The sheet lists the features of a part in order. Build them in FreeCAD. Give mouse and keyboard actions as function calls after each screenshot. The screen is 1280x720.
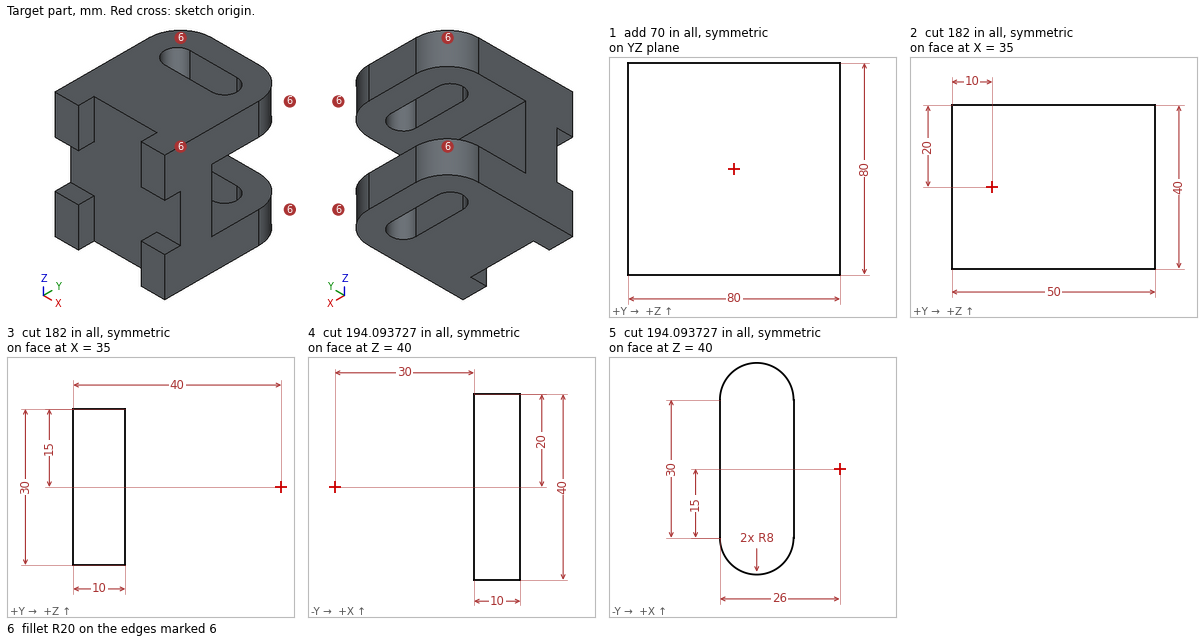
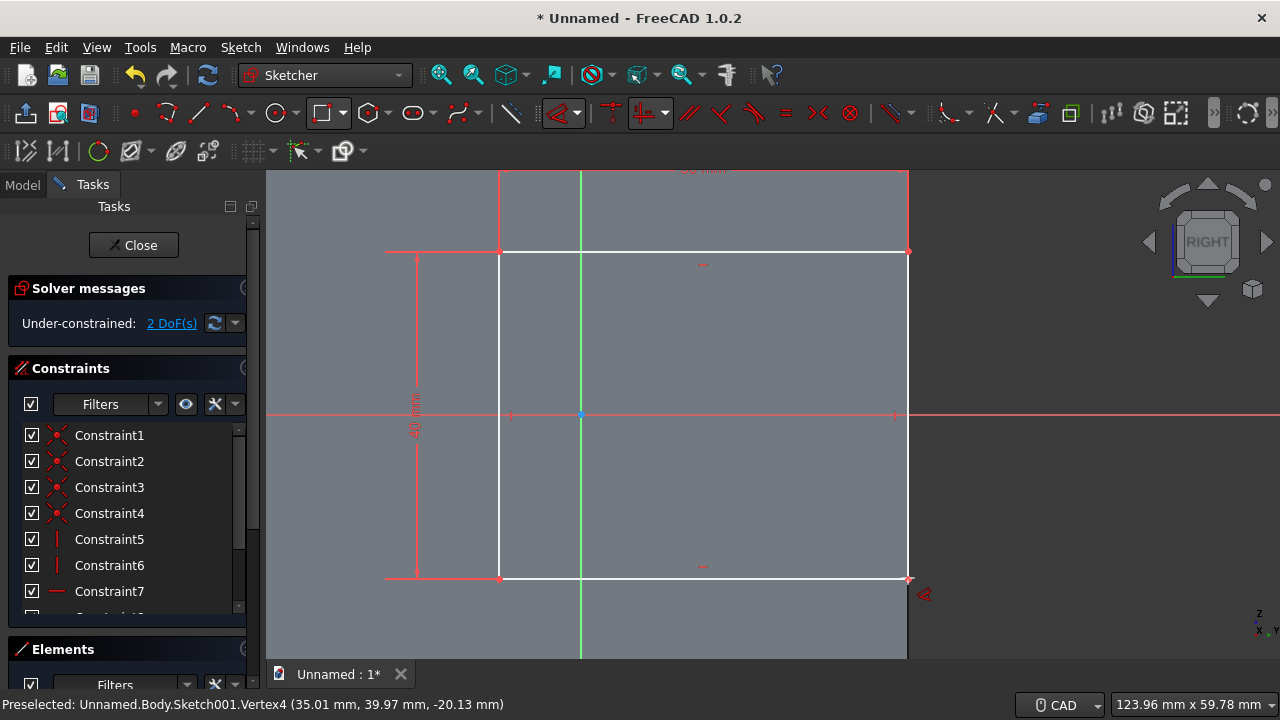
click(499, 252)
click(540, 218)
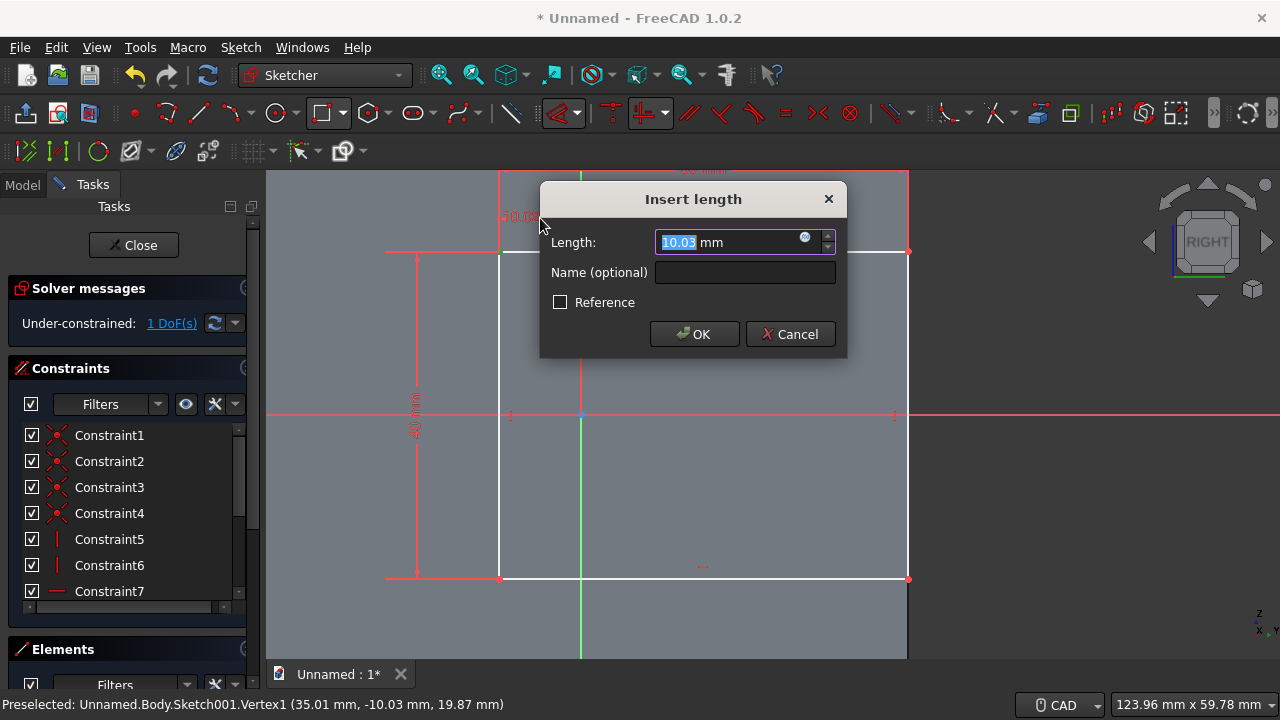
text(10)
key(Return)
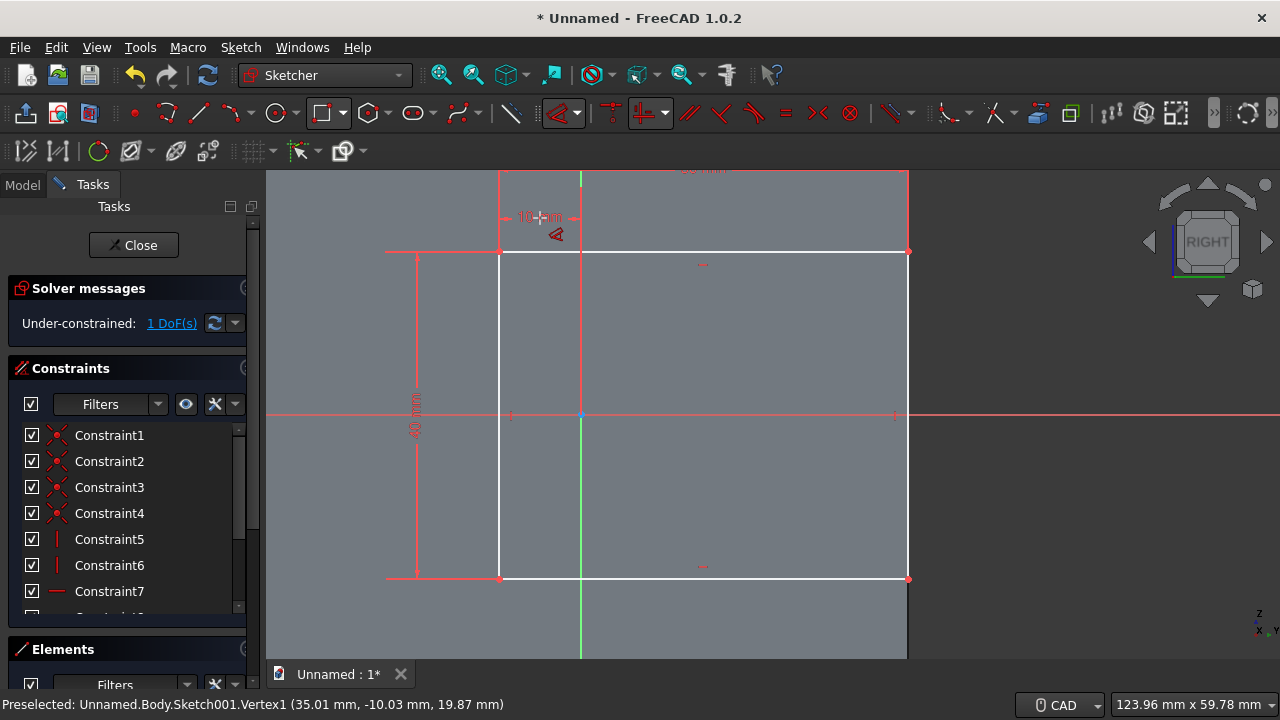
click(499, 252)
click(465, 333)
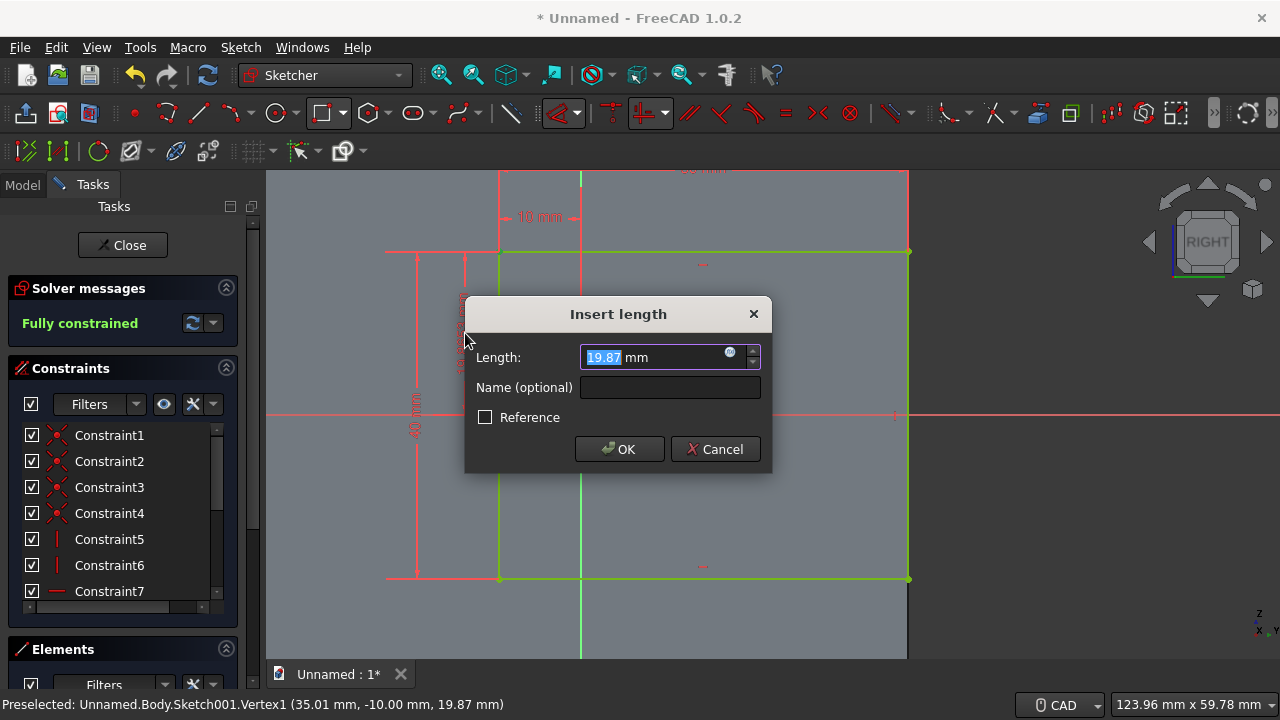
text(20)
key(Return)
key(Escape)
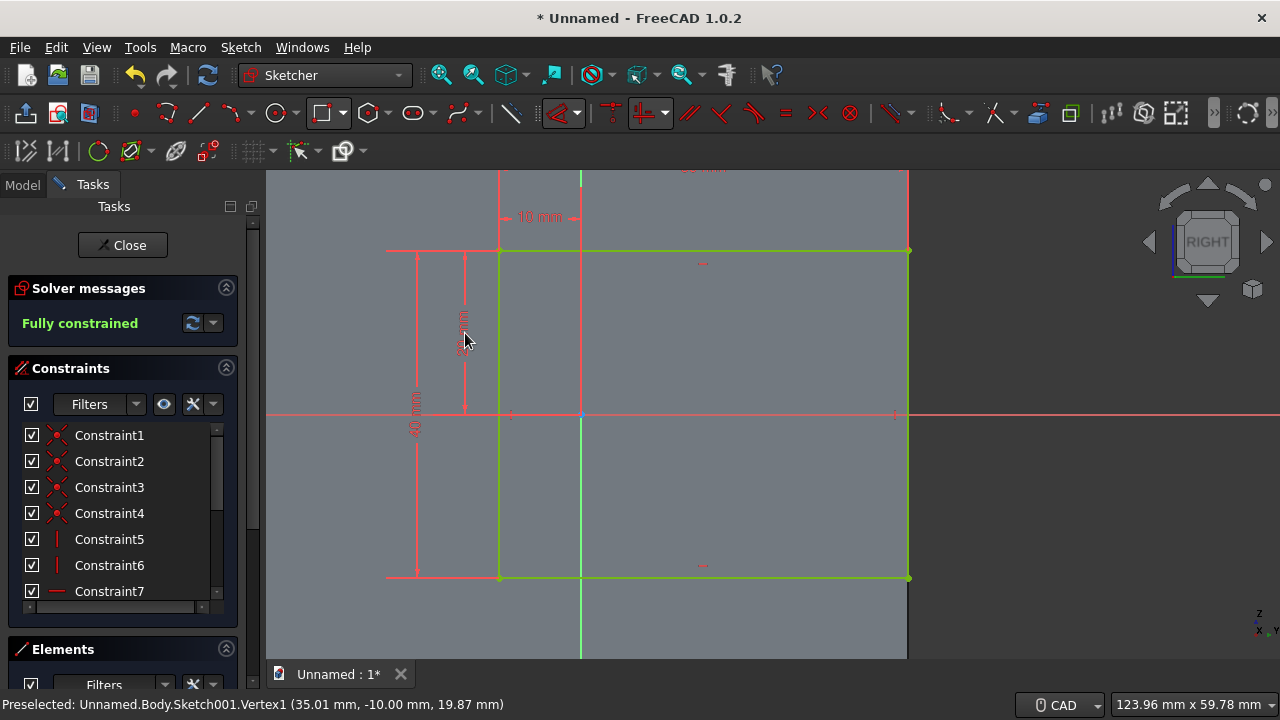
click(123, 245)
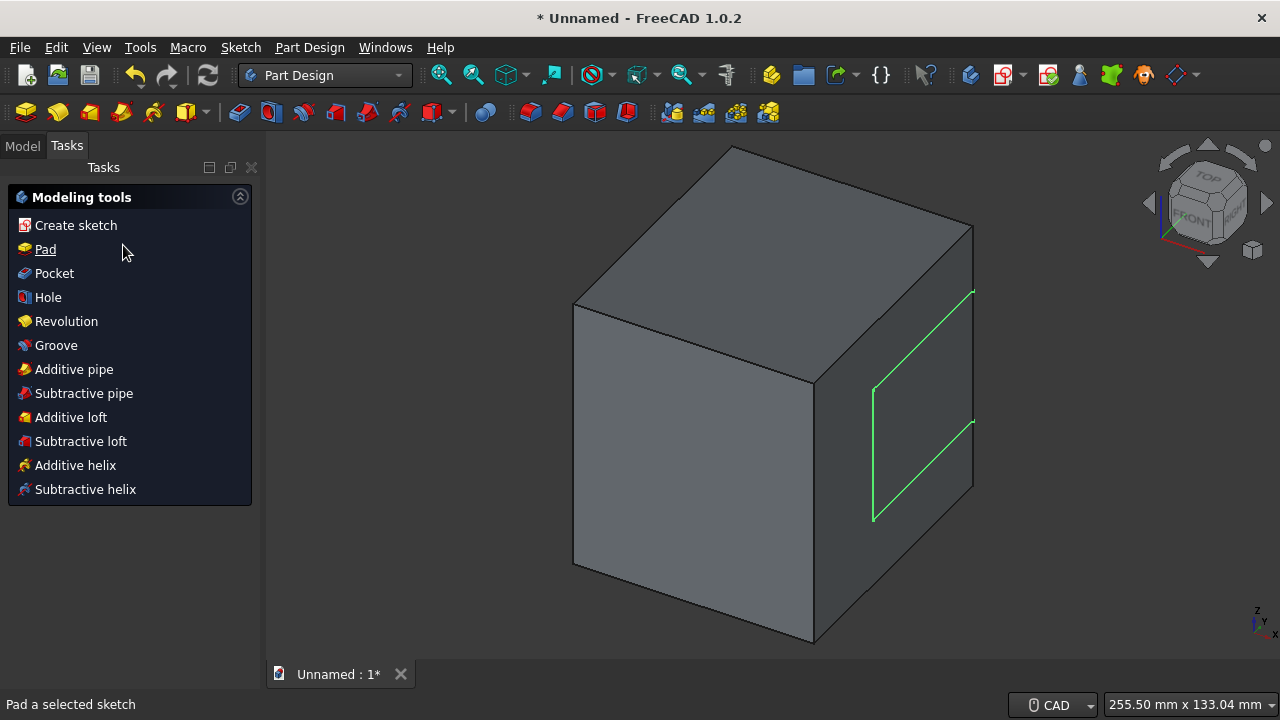
click(240, 112)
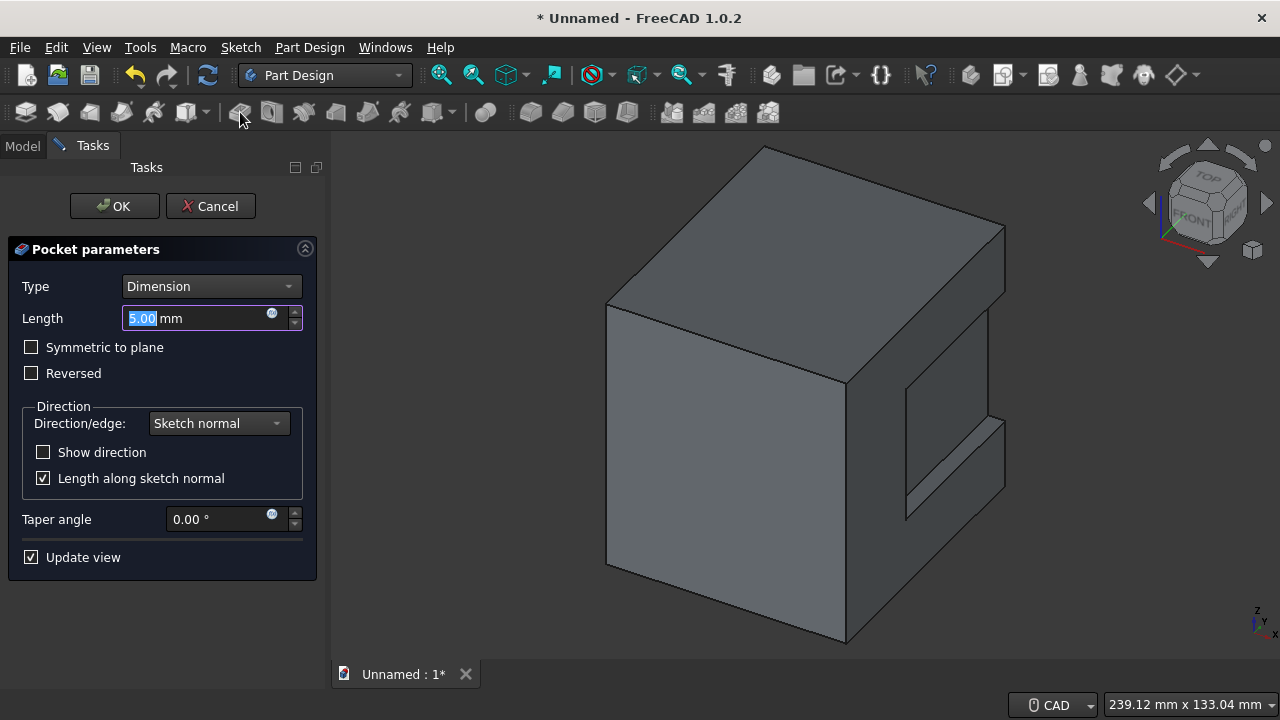
text(182)
key(Tab)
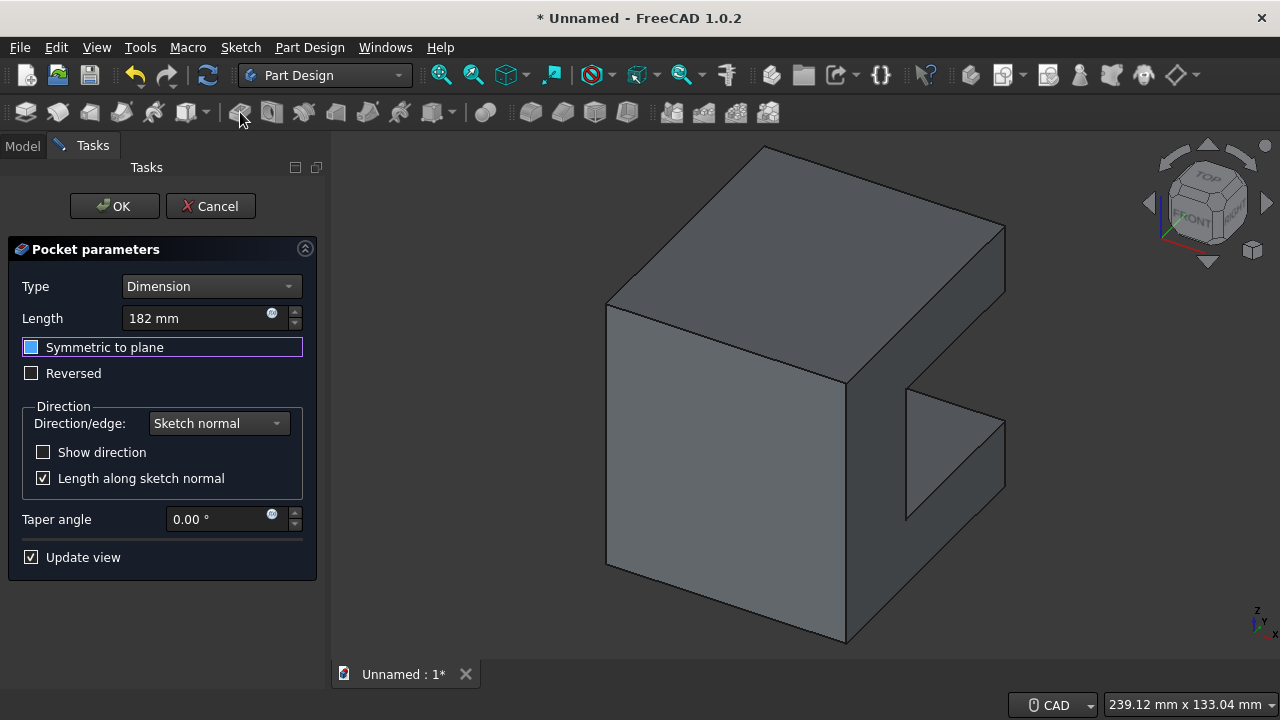
click(30, 347)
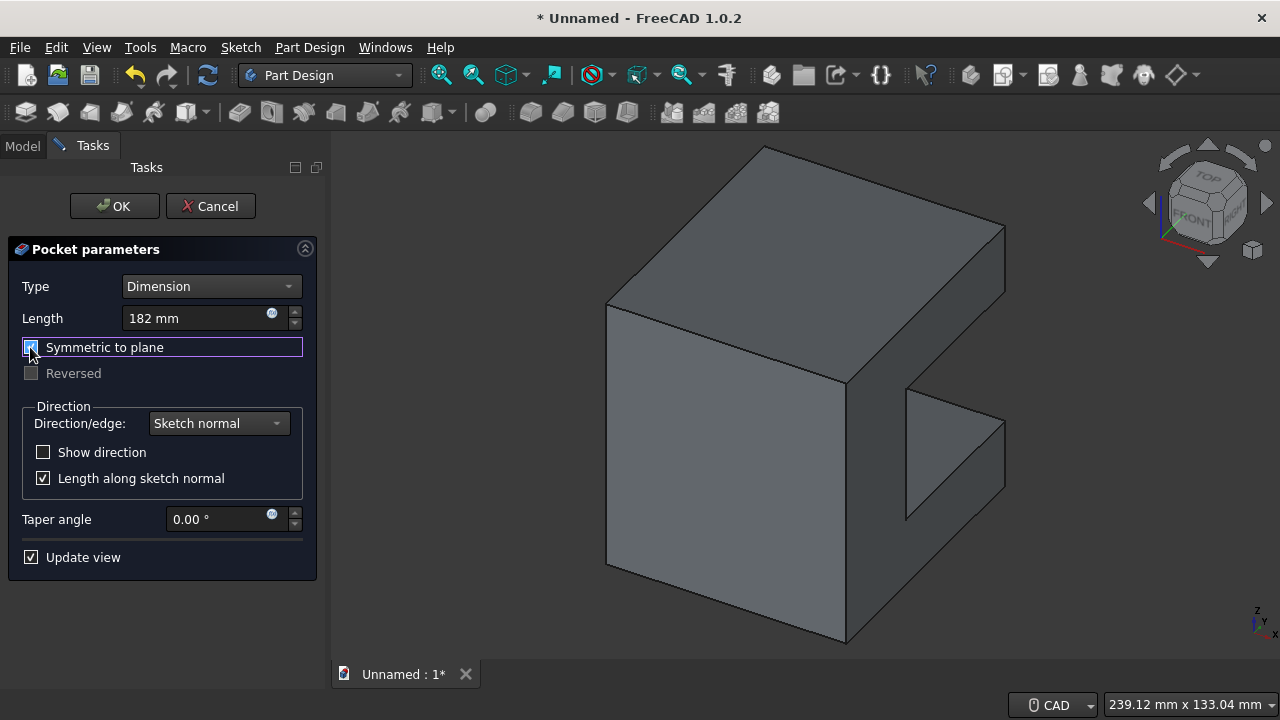
click(115, 206)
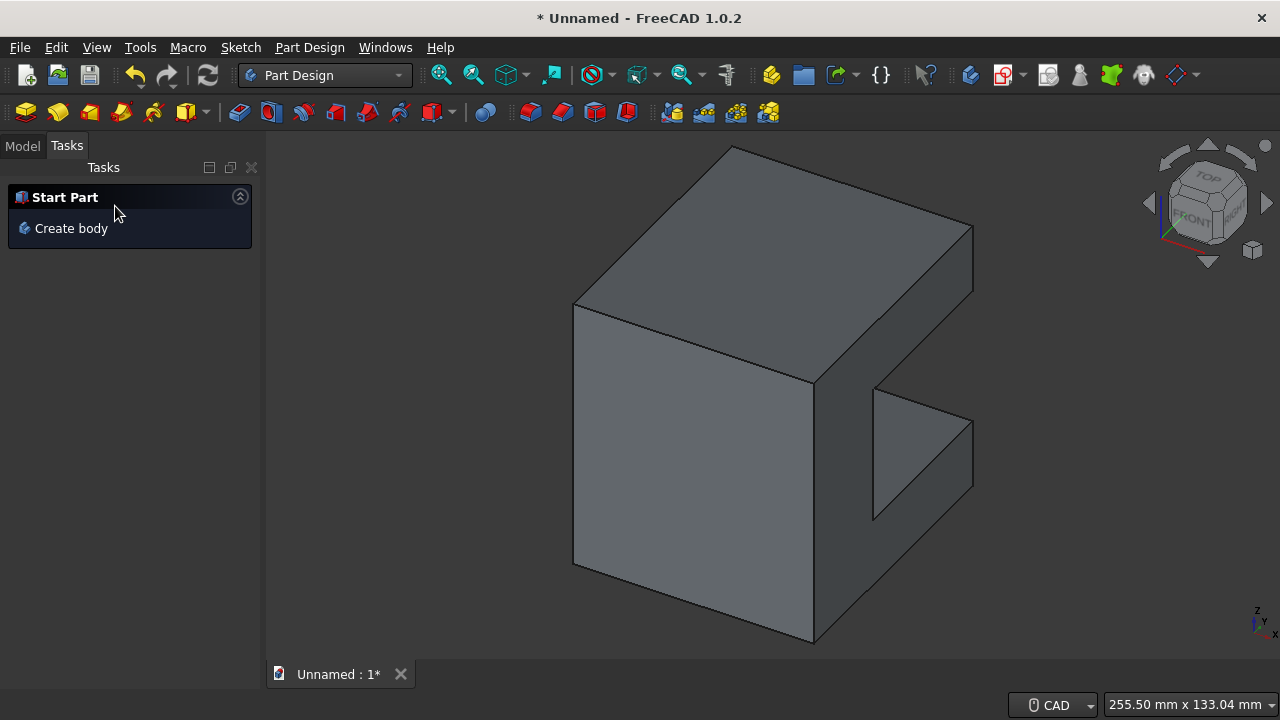
click(848, 553)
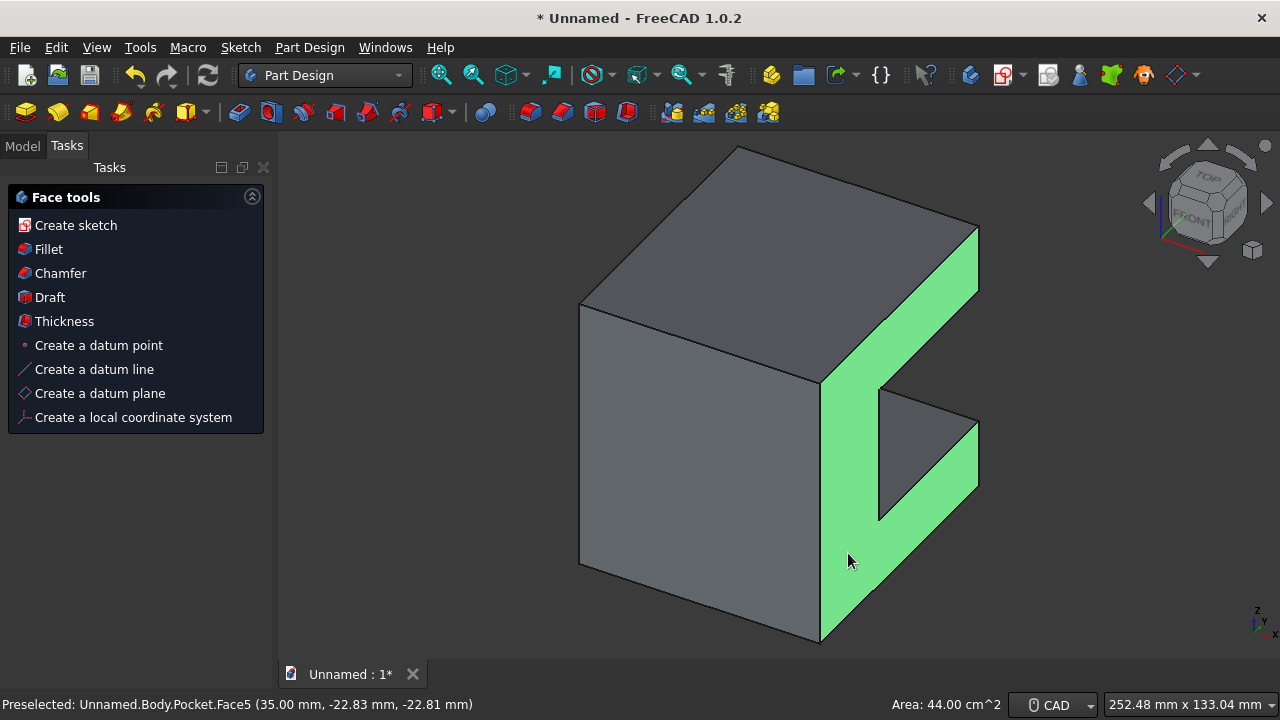
click(1004, 76)